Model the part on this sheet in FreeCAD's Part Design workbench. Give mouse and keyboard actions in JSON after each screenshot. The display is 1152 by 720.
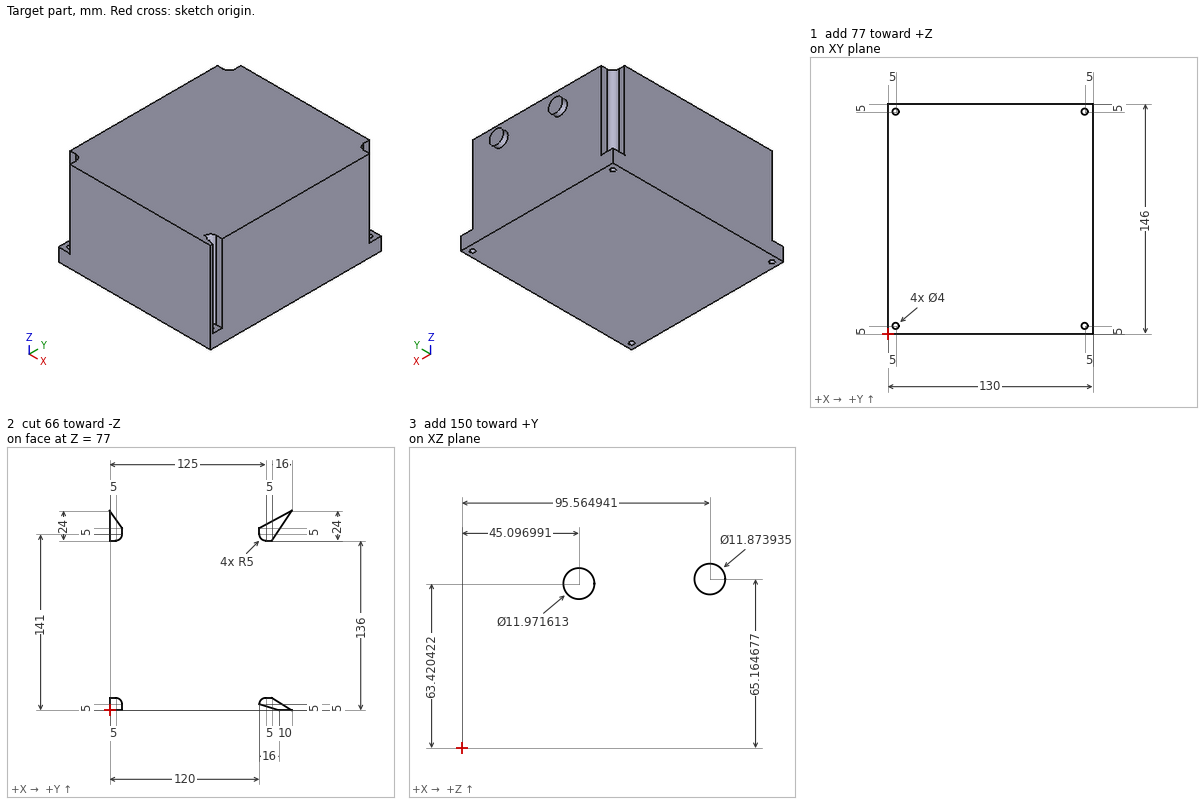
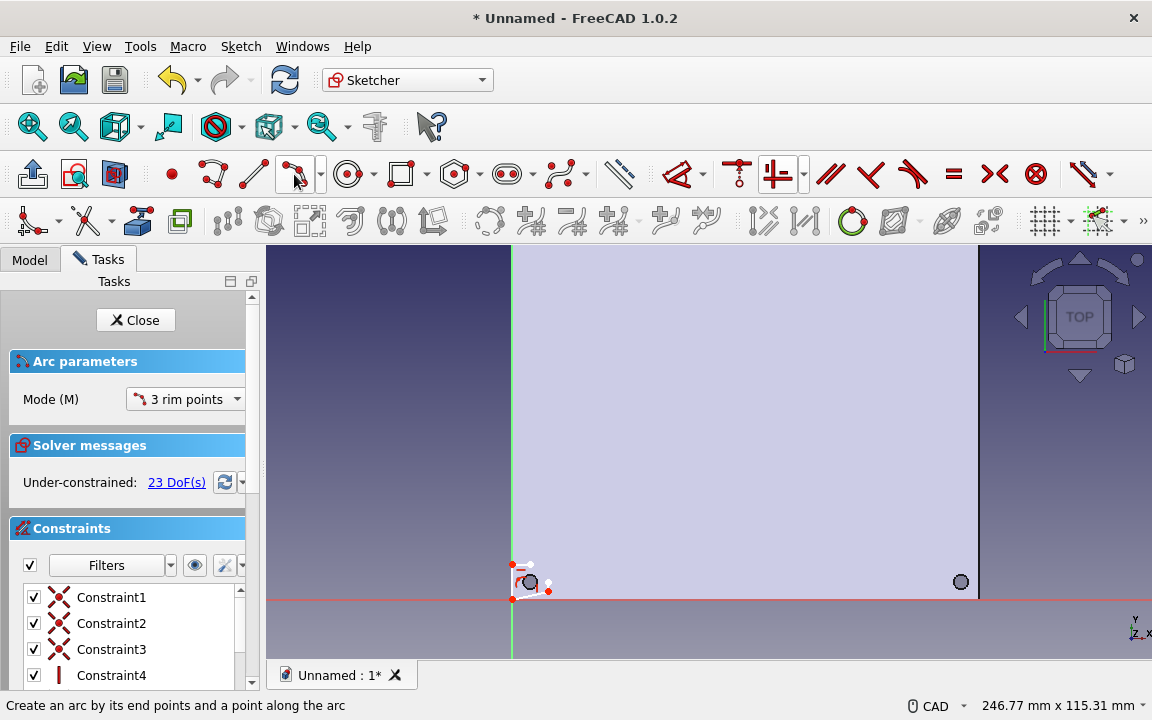
{"action": "scroll", "coordinate": [548, 582], "scroll_direction": "up", "scroll_amount": 3}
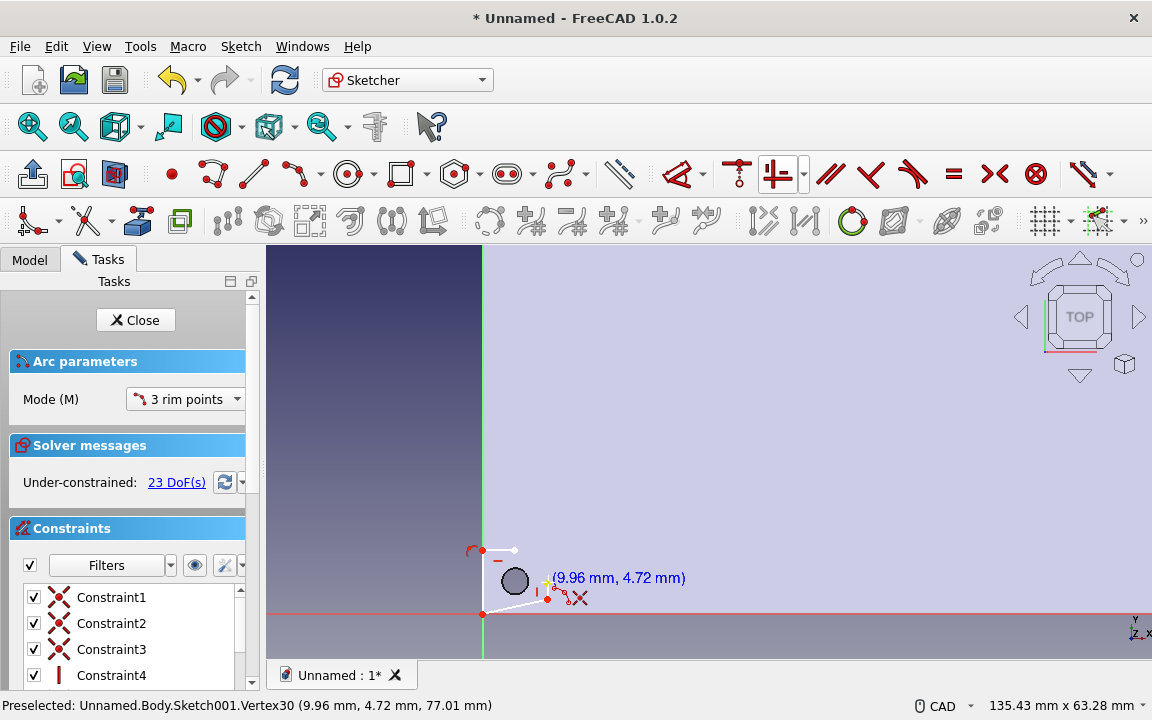
{"action": "left_click", "coordinate": [548, 583]}
{"action": "left_click", "coordinate": [515, 550]}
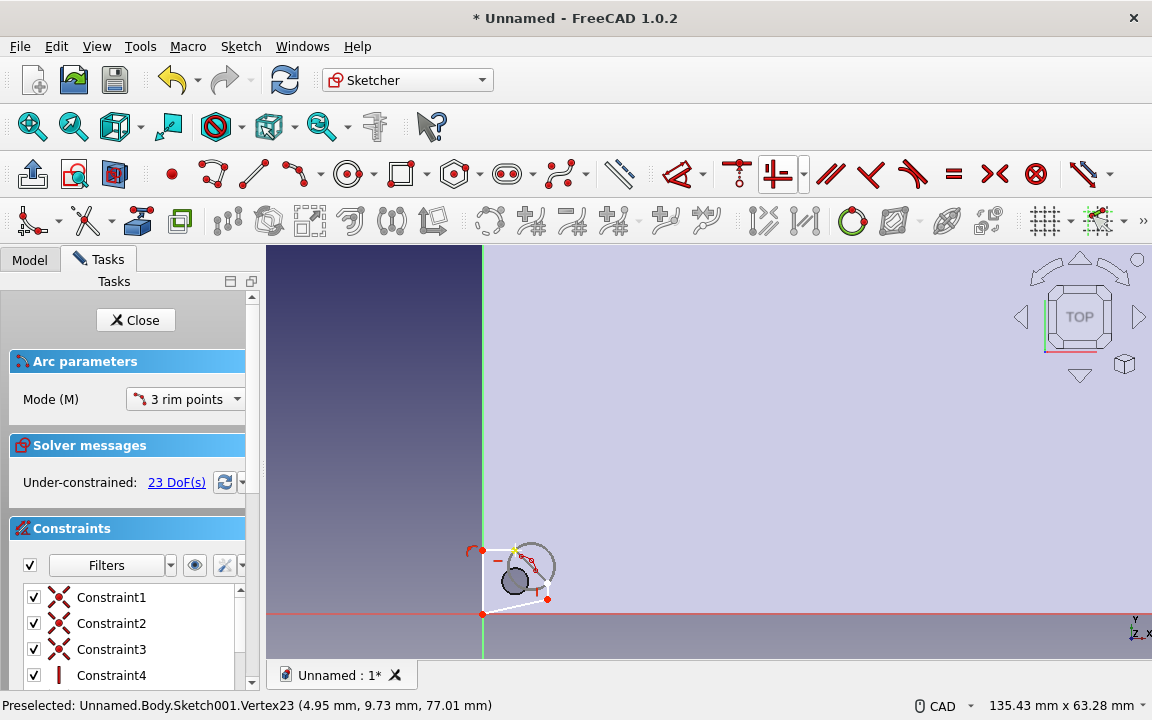
{"action": "scroll", "coordinate": [538, 558], "scroll_direction": "up", "scroll_amount": 3}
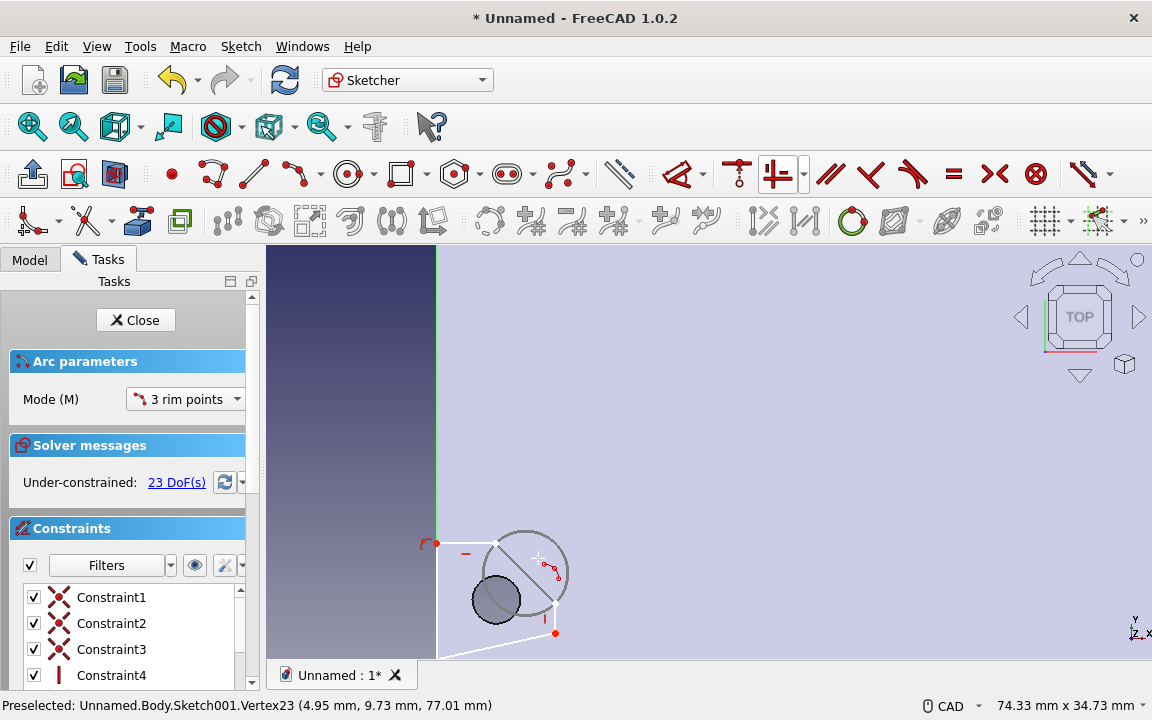
{"action": "left_click", "coordinate": [538, 558]}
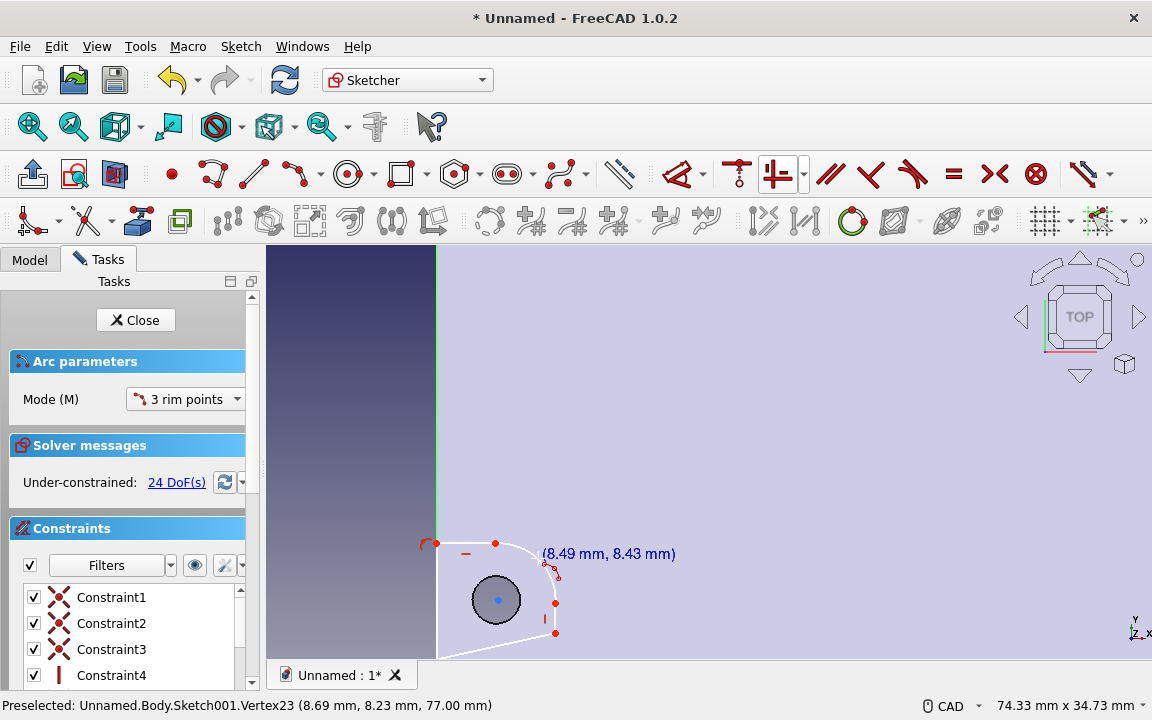
{"action": "left_click", "coordinate": [213, 174]}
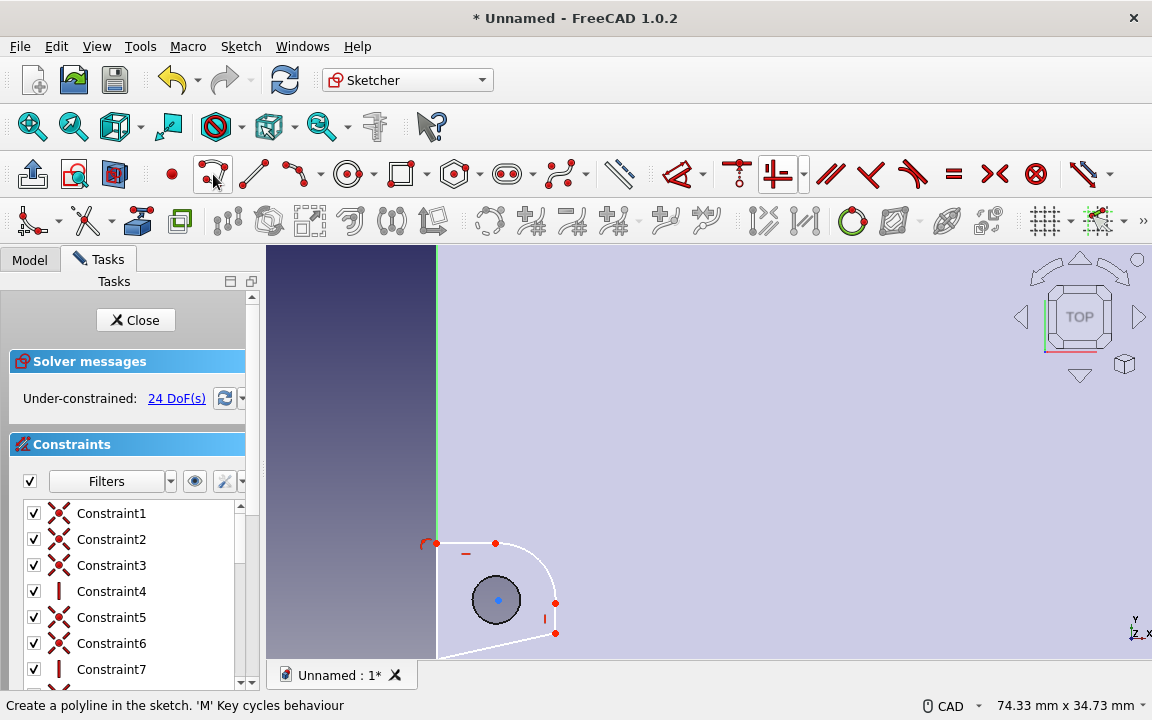
{"action": "scroll", "coordinate": [536, 569], "scroll_direction": "down", "scroll_amount": 10}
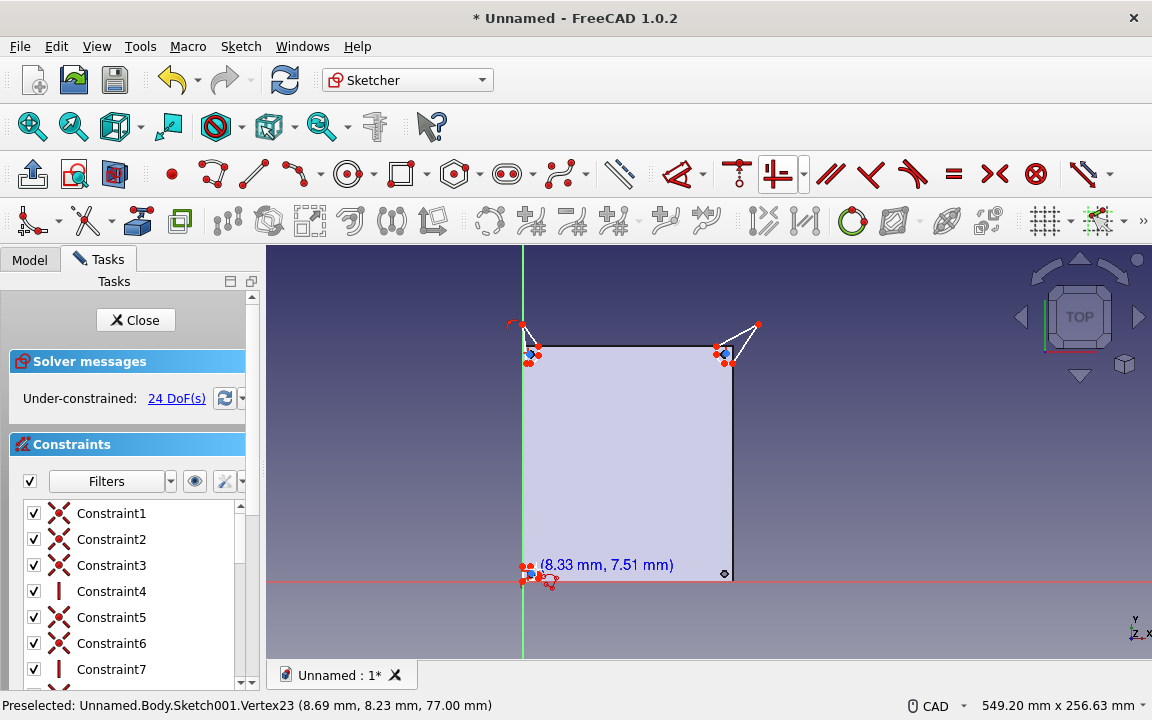
{"action": "scroll", "coordinate": [716, 574], "scroll_direction": "up", "scroll_amount": 4}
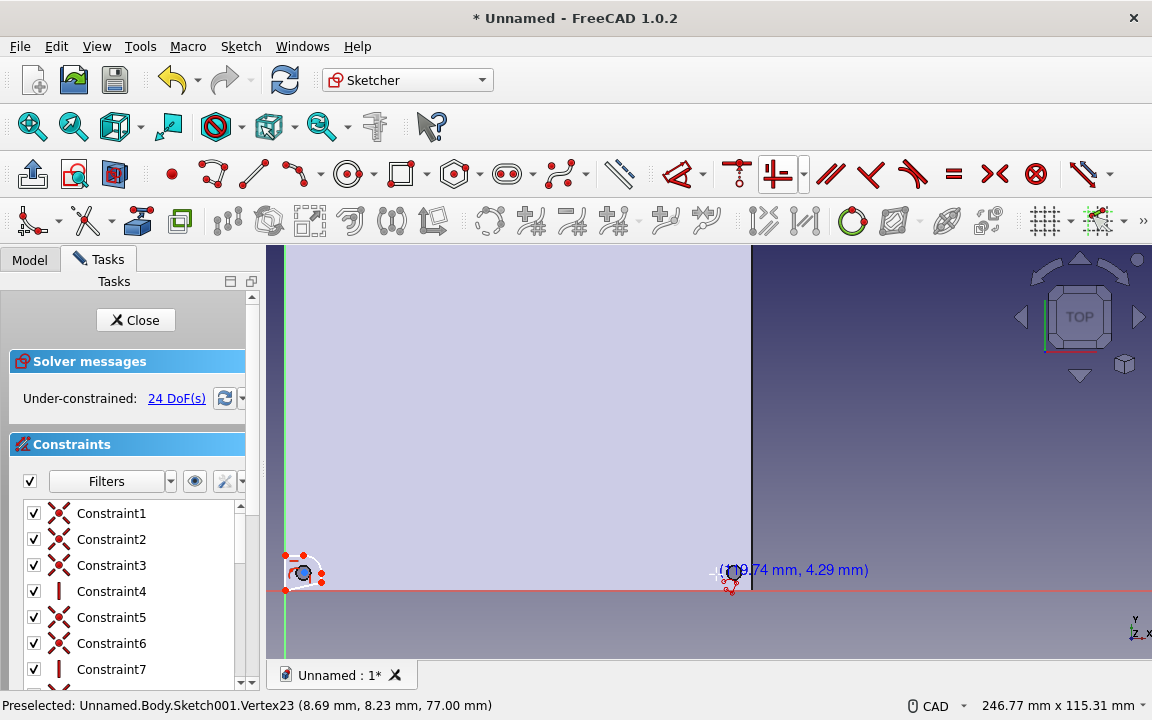
{"action": "left_click", "coordinate": [716, 573]}
{"action": "left_click", "coordinate": [774, 591]}
{"action": "left_click", "coordinate": [810, 582]}
{"action": "left_click", "coordinate": [752, 555]}
{"action": "left_click", "coordinate": [734, 555]}
{"action": "right_click", "coordinate": [734, 555]}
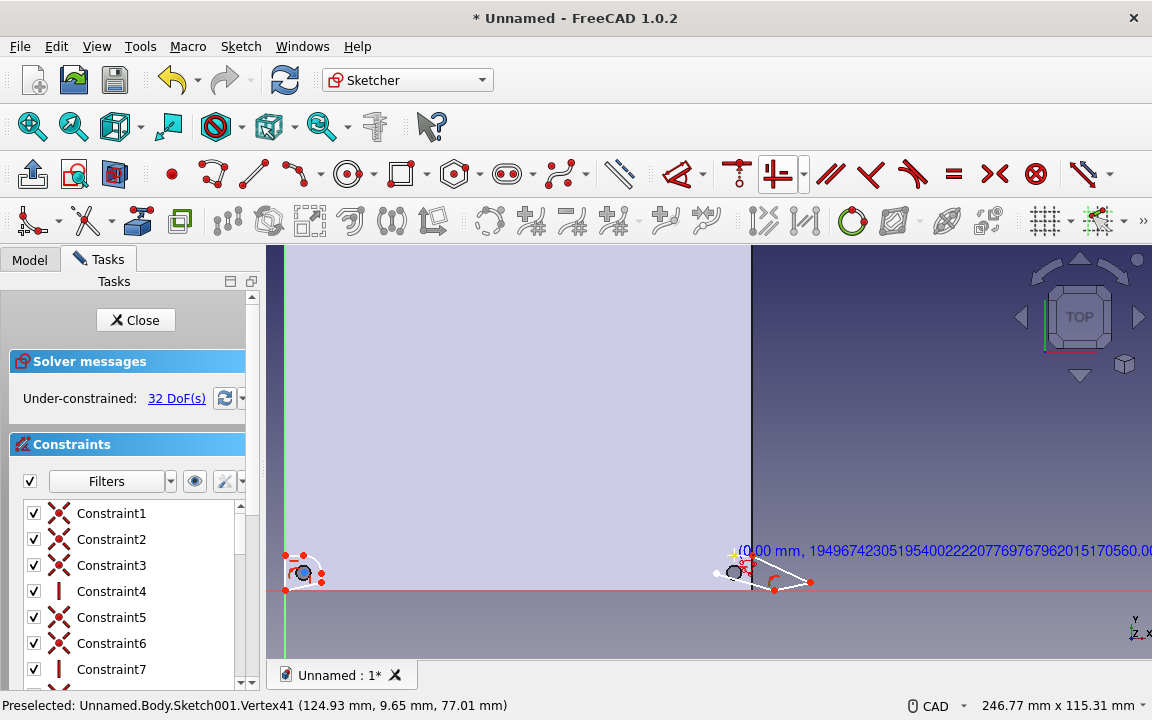
{"action": "left_click", "coordinate": [294, 174]}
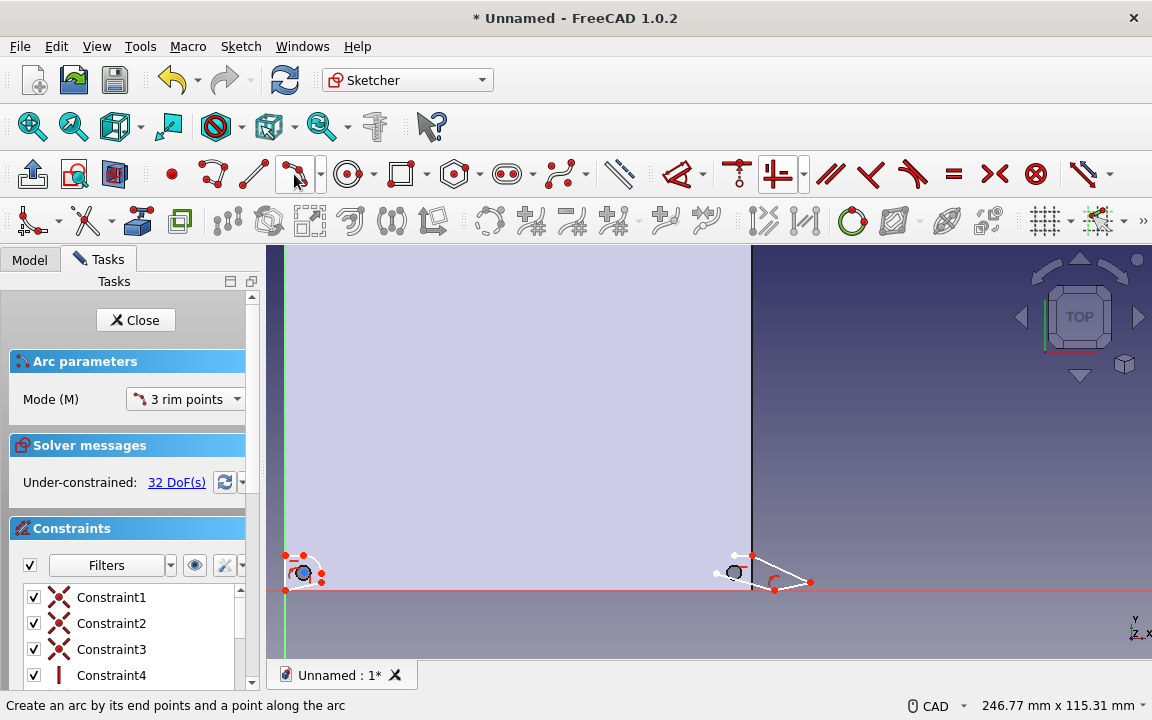
{"action": "scroll", "coordinate": [734, 555], "scroll_direction": "up", "scroll_amount": 3}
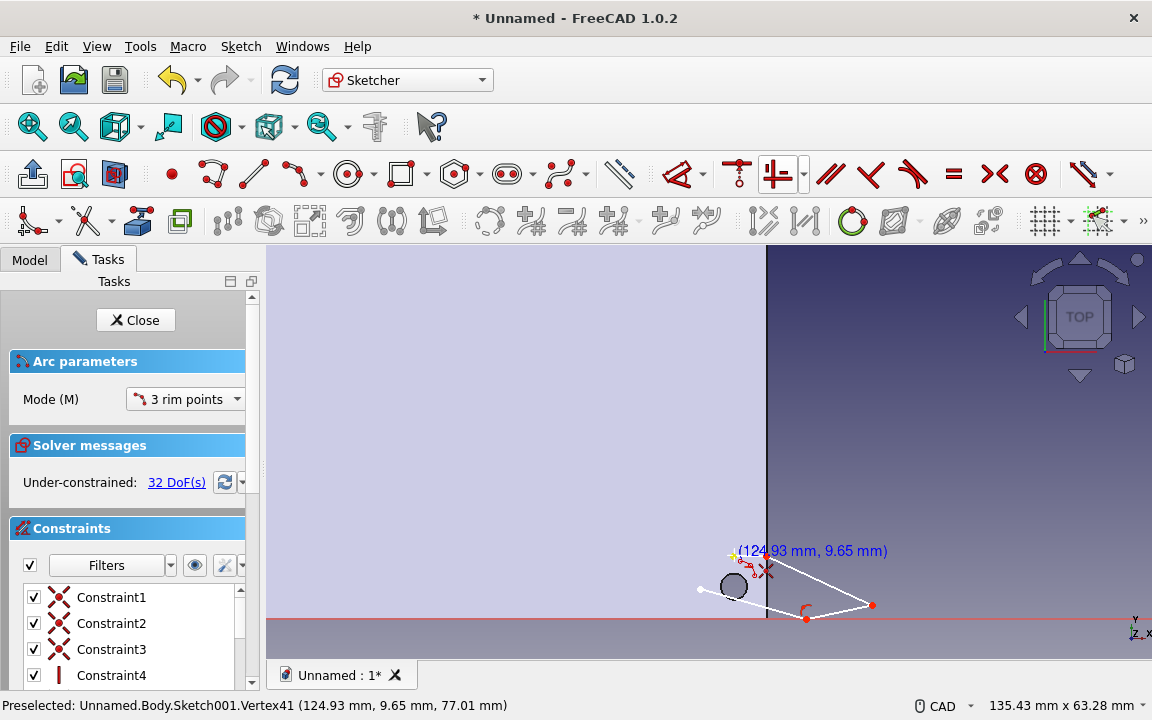
{"action": "left_click", "coordinate": [734, 556]}
{"action": "left_click", "coordinate": [701, 589]}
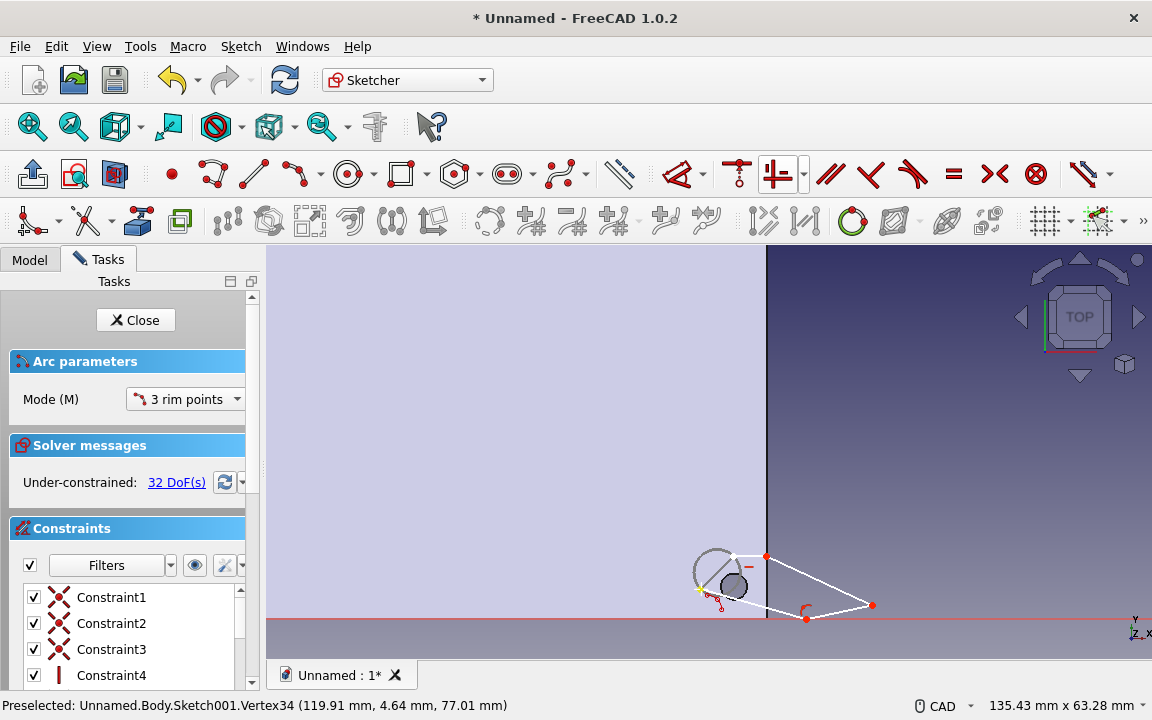
{"action": "scroll", "coordinate": [711, 564], "scroll_direction": "up", "scroll_amount": 3}